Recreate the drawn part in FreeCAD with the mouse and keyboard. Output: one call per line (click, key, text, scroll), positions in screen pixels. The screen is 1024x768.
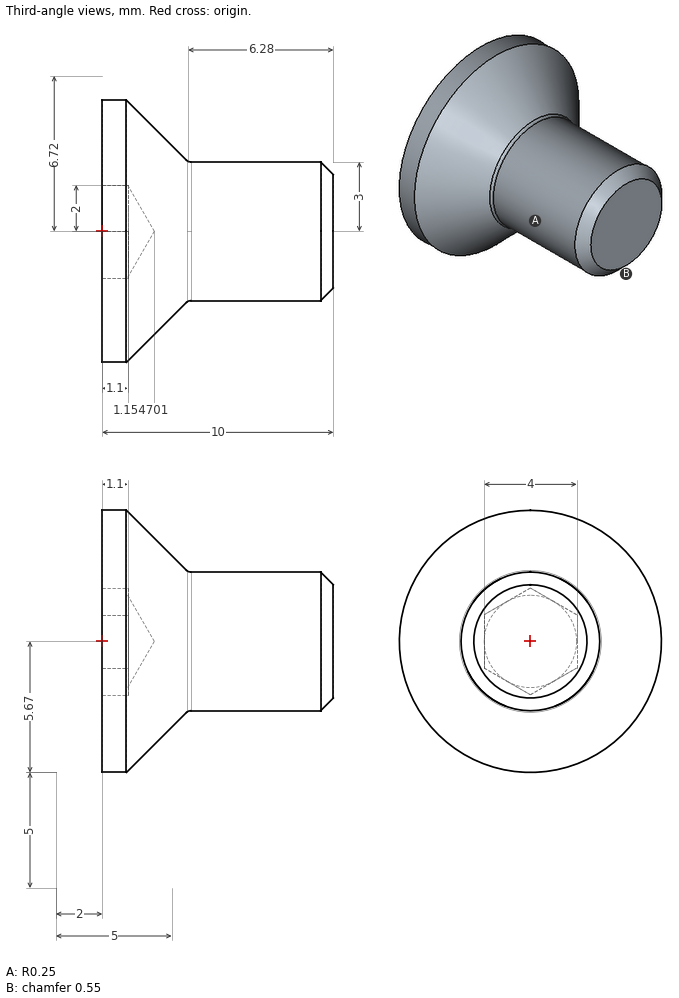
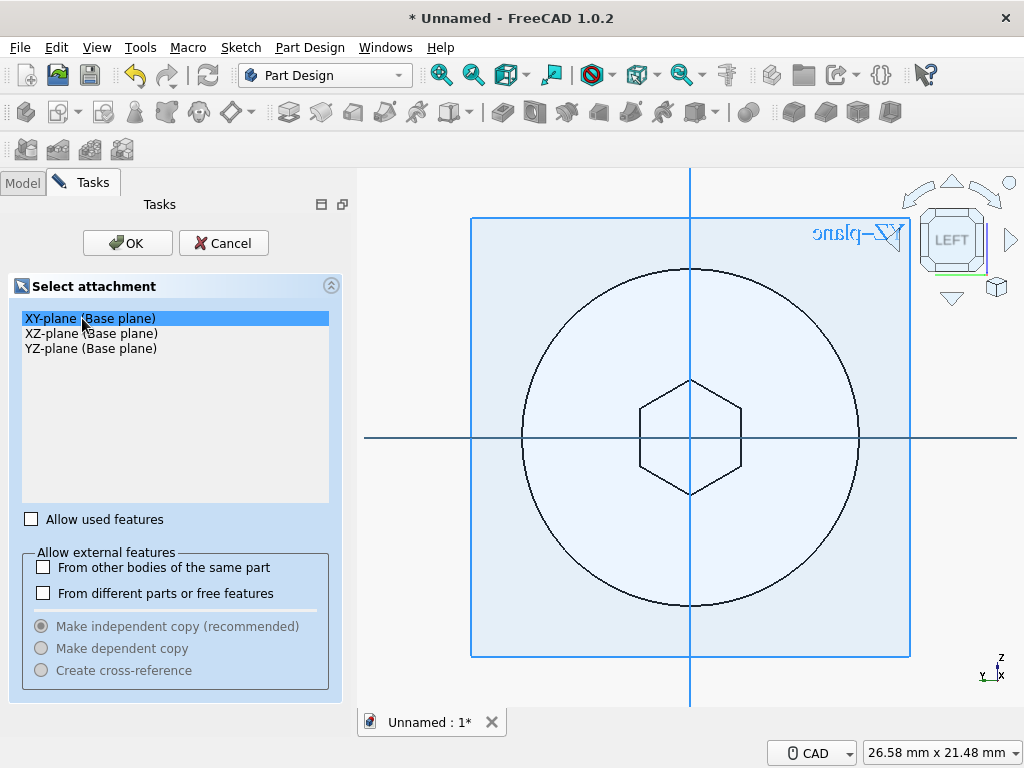
click(128, 243)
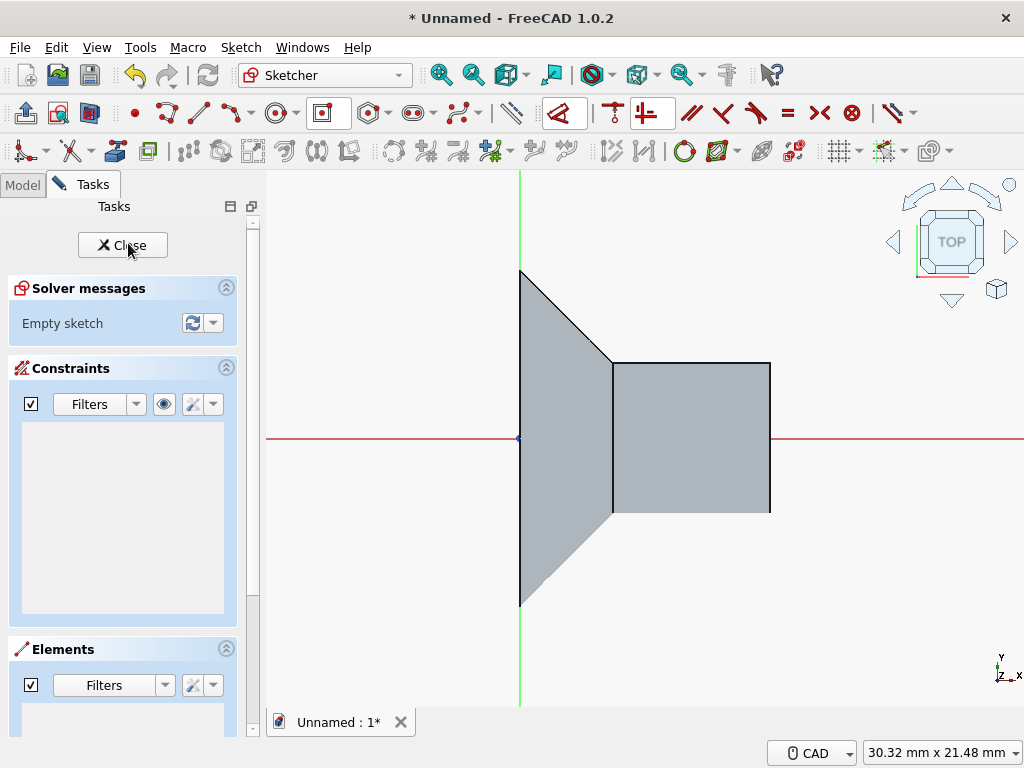
key(q)
key(s)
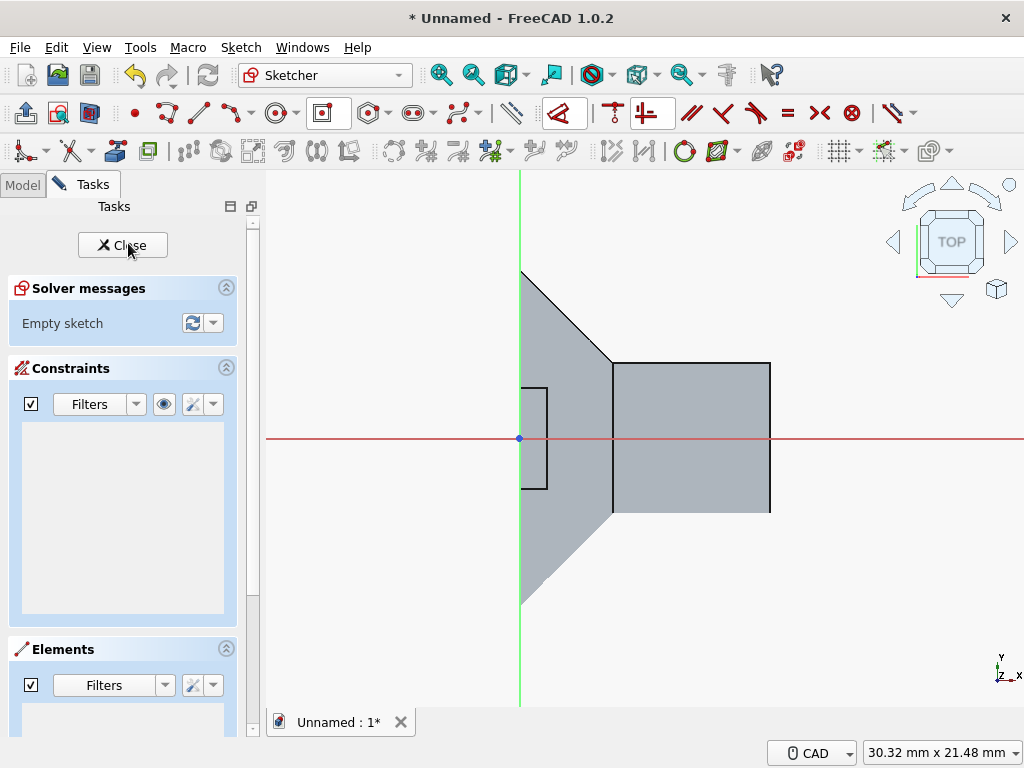
scroll(544, 410, up, 10)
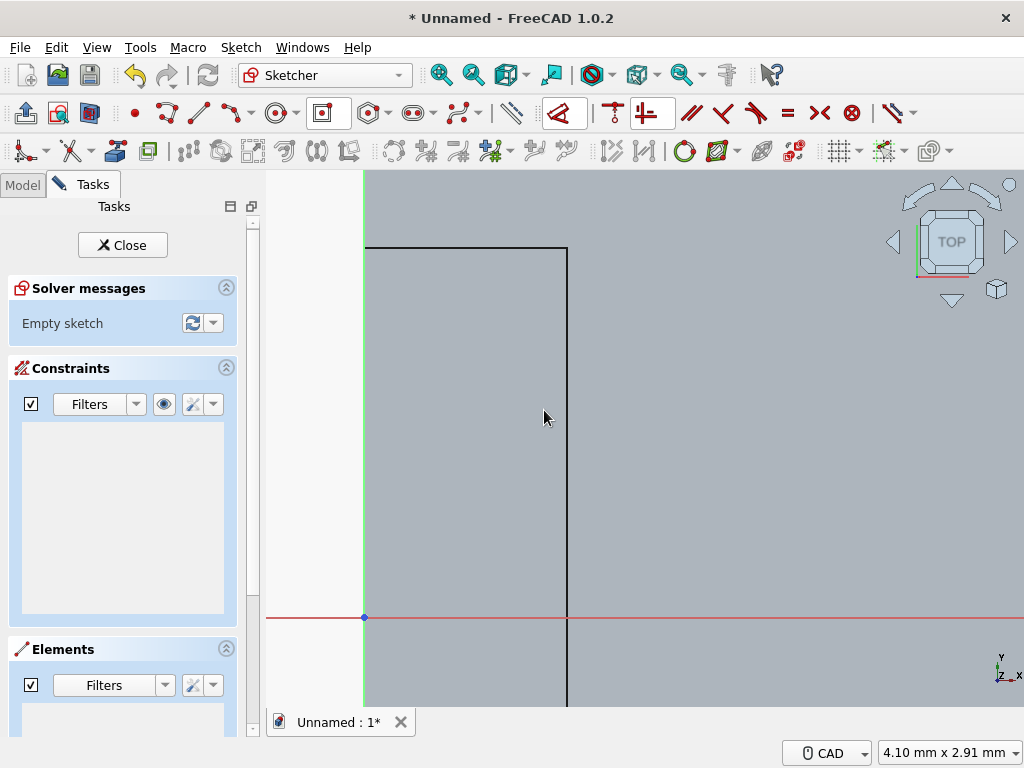
key(g)
key(m)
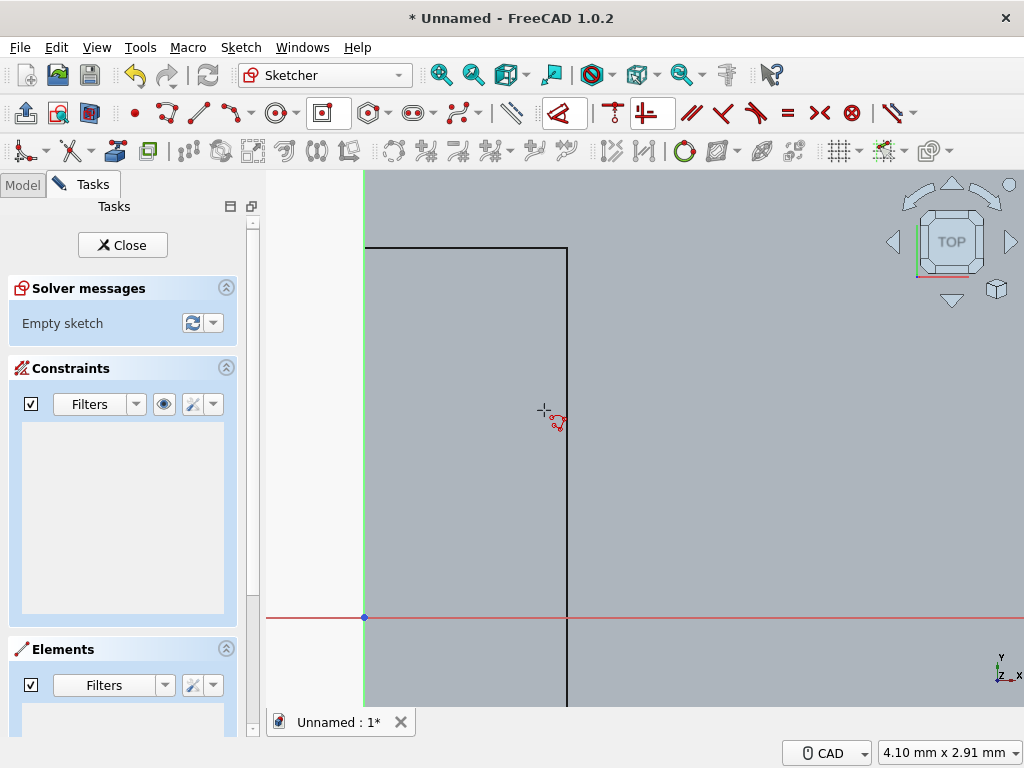
click(567, 618)
click(781, 609)
click(567, 248)
click(567, 618)
key(Escape)
key(Escape)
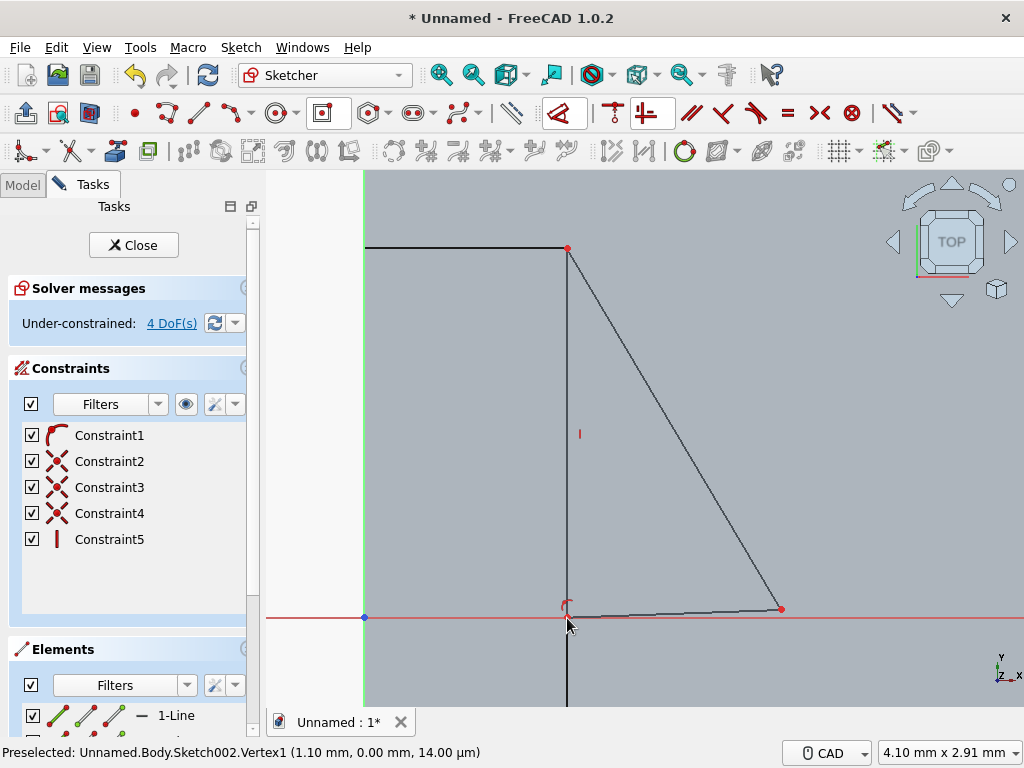
click(631, 615)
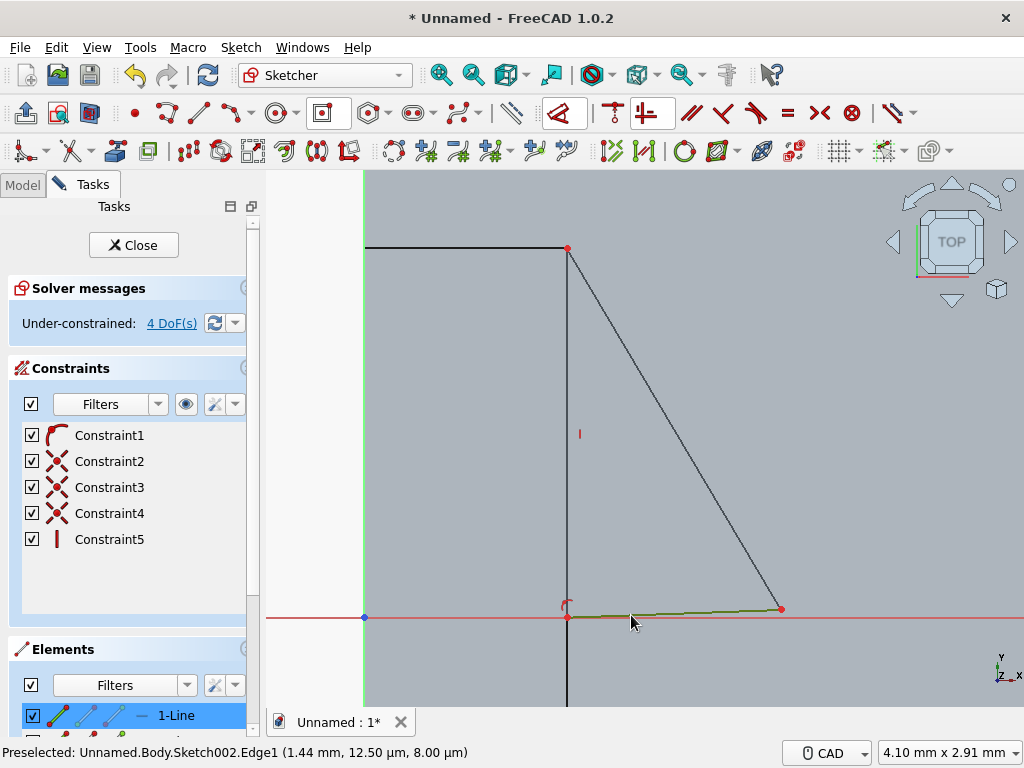
key(h)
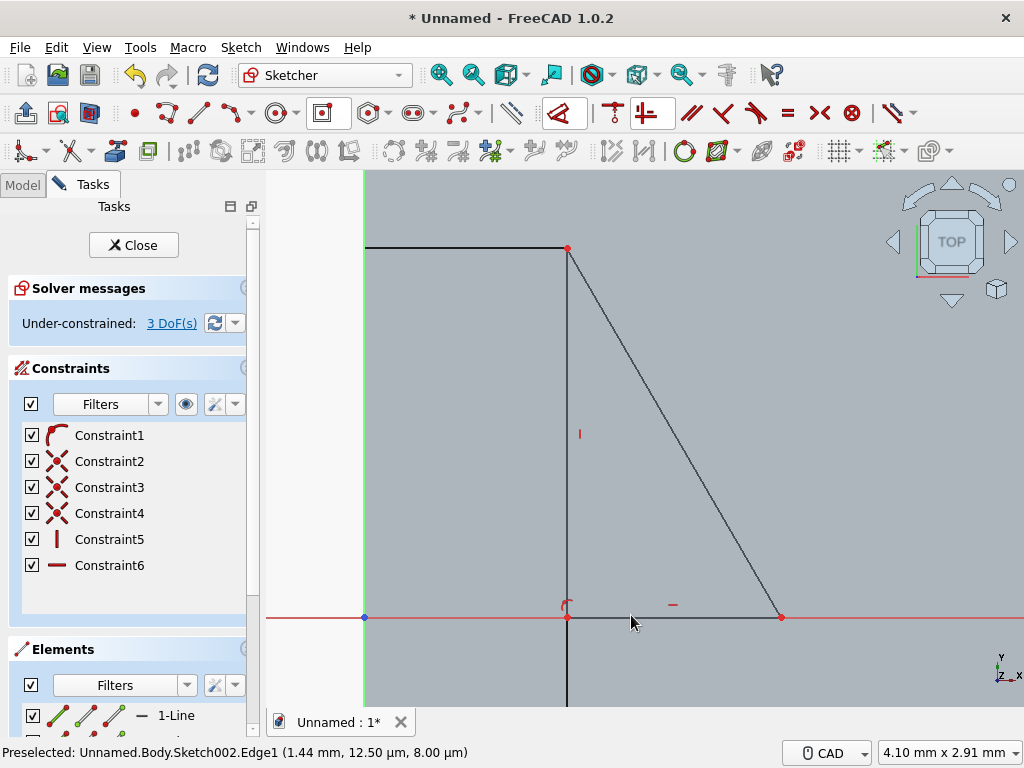
click(558, 114)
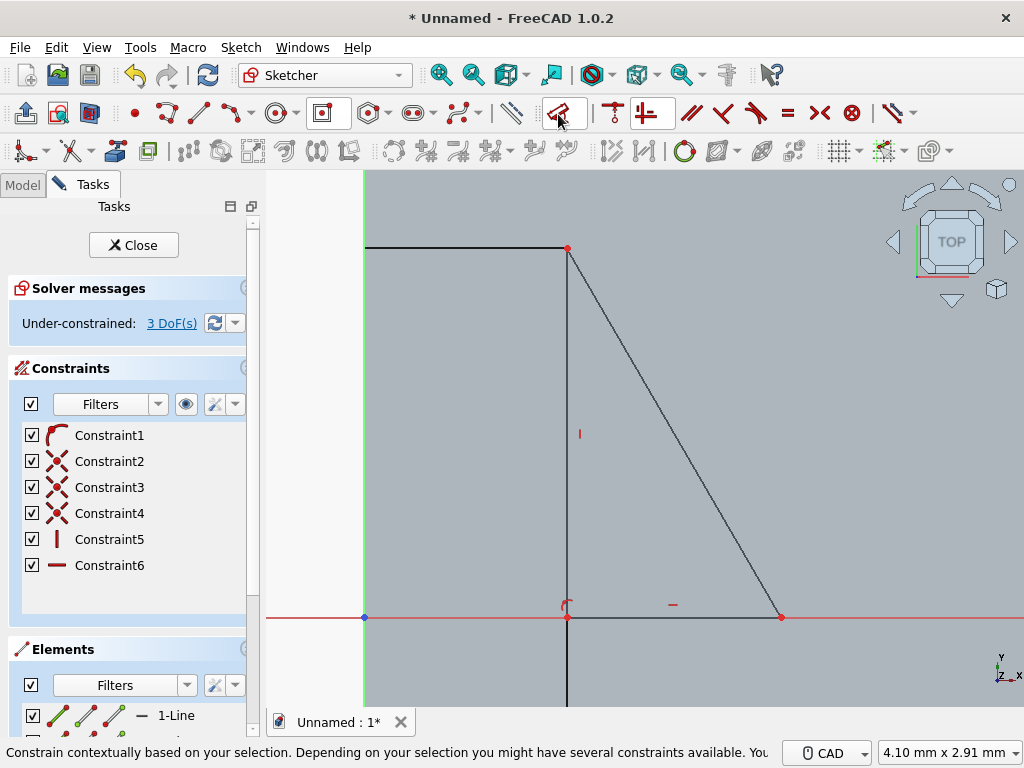
click(567, 360)
click(533, 433)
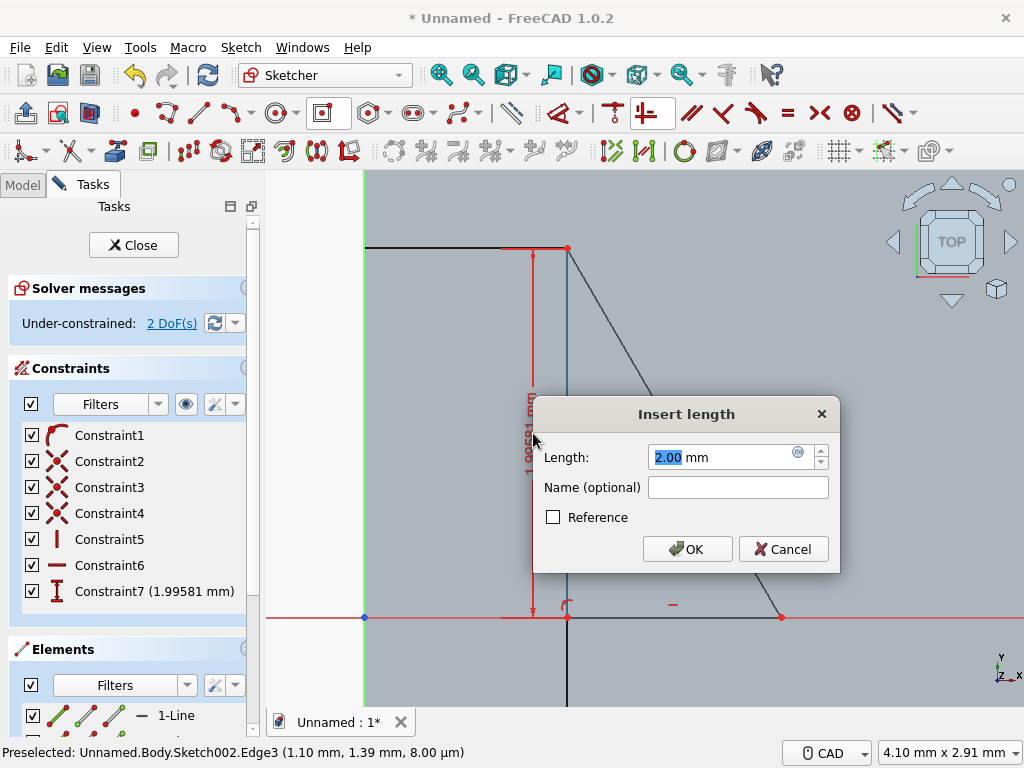
text(2)
key(Return)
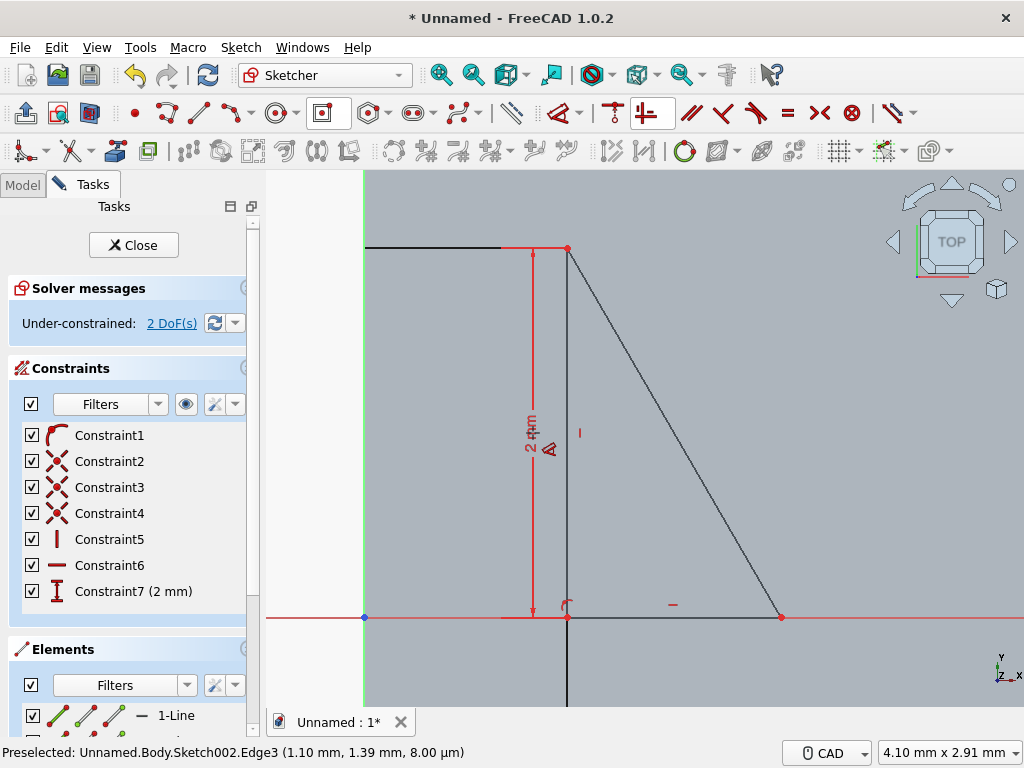
click(567, 618)
click(466, 652)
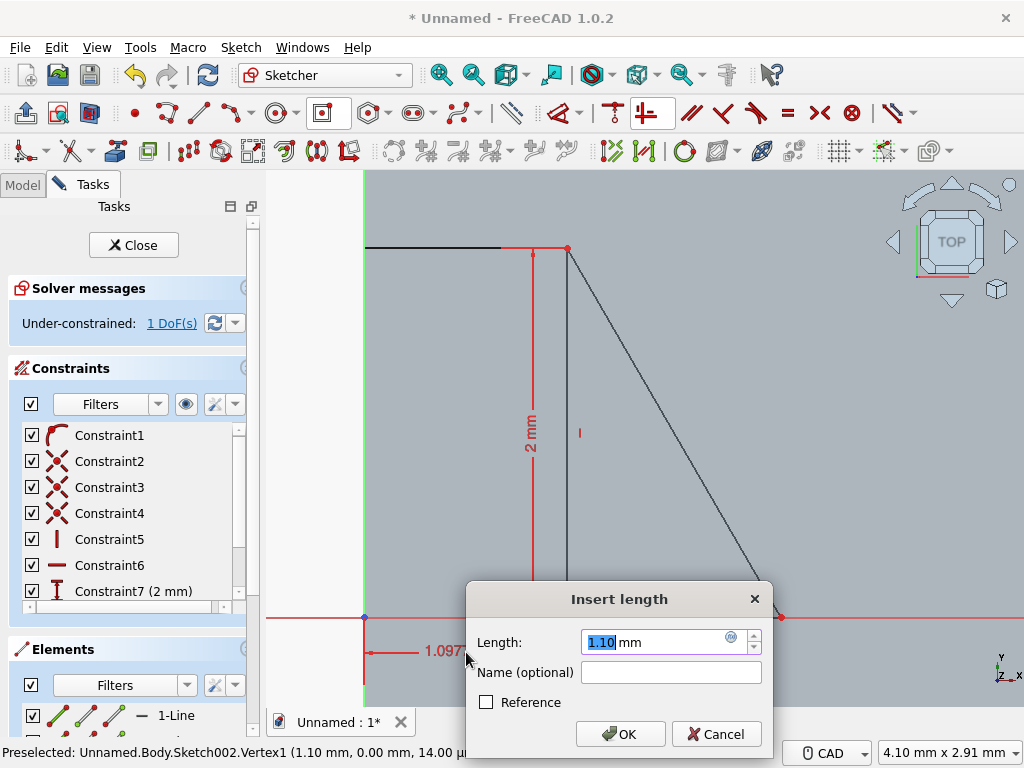
text(1.1)
key(Return)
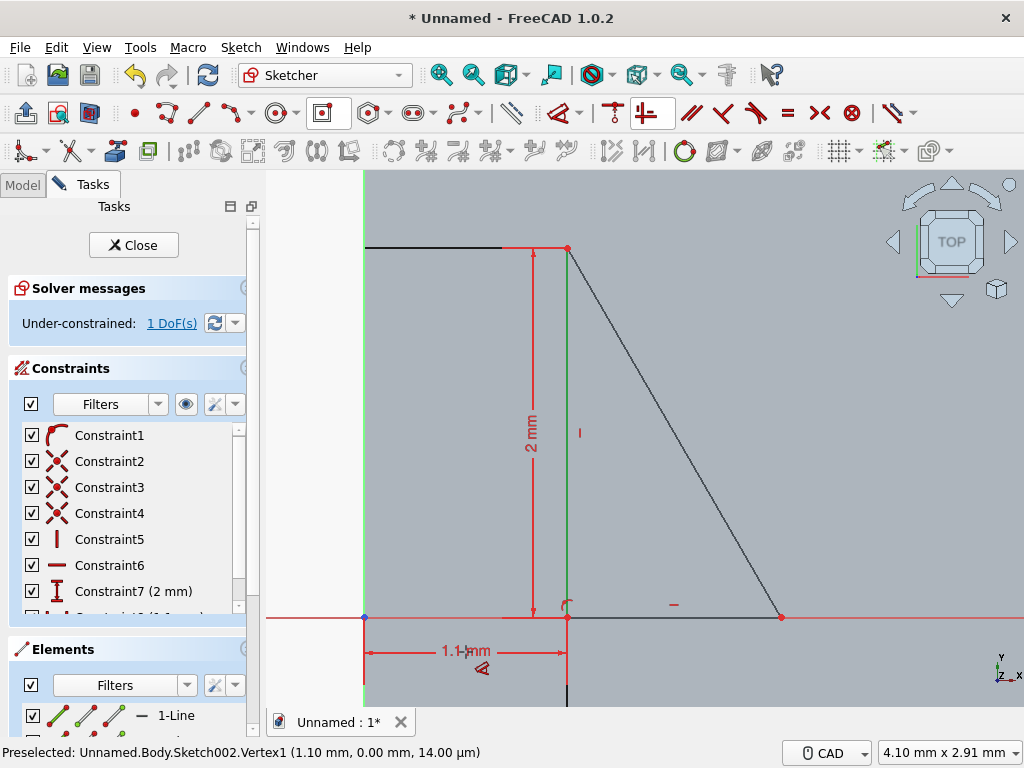
click(631, 618)
click(674, 652)